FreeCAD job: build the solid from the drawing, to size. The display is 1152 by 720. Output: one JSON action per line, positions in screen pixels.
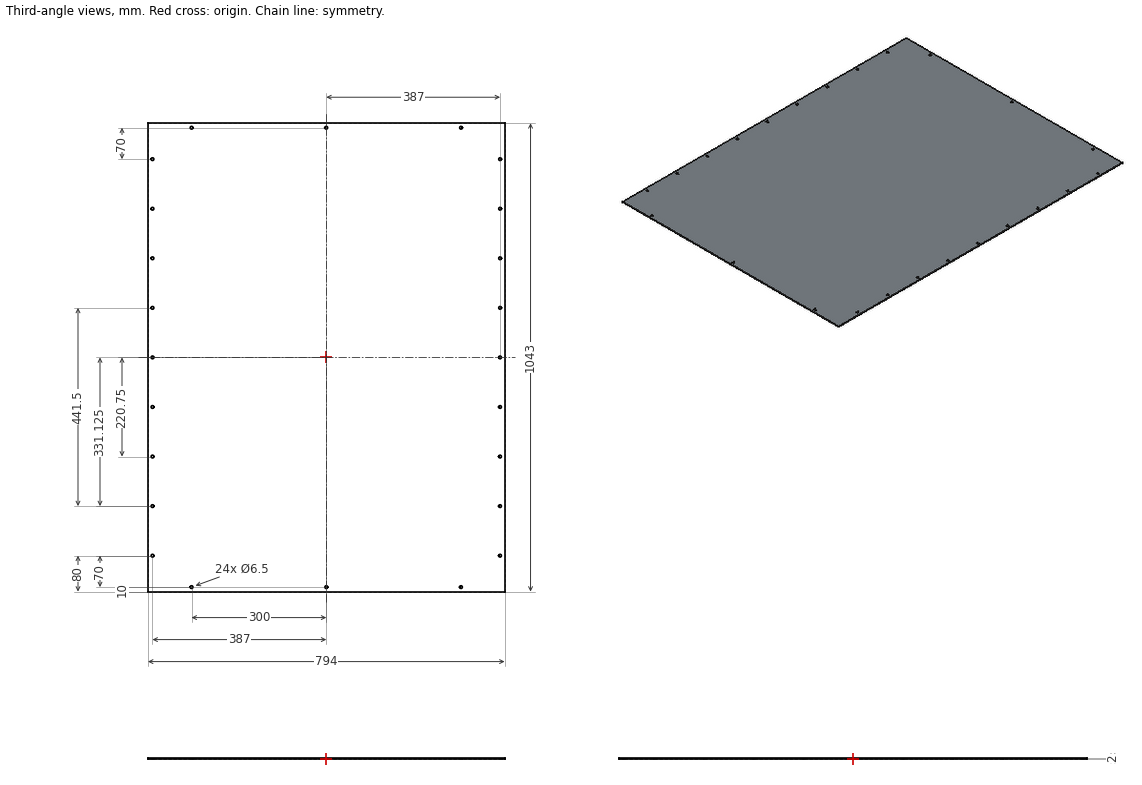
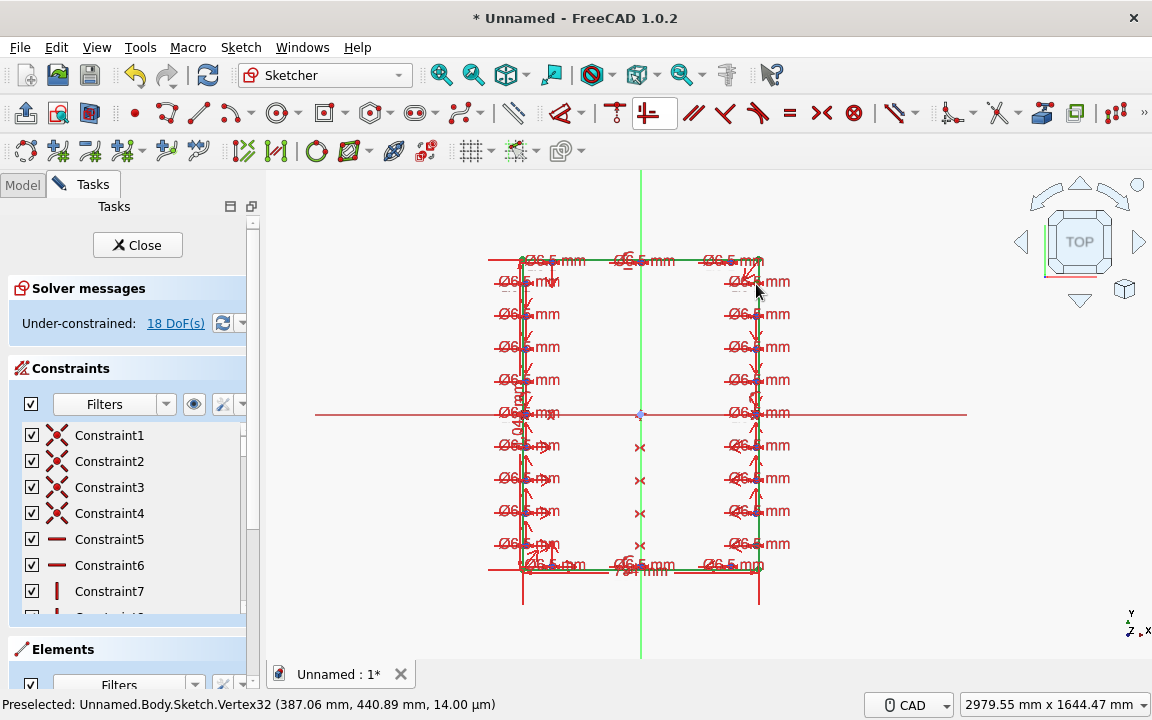
{"action": "left_click", "coordinate": [344, 415]}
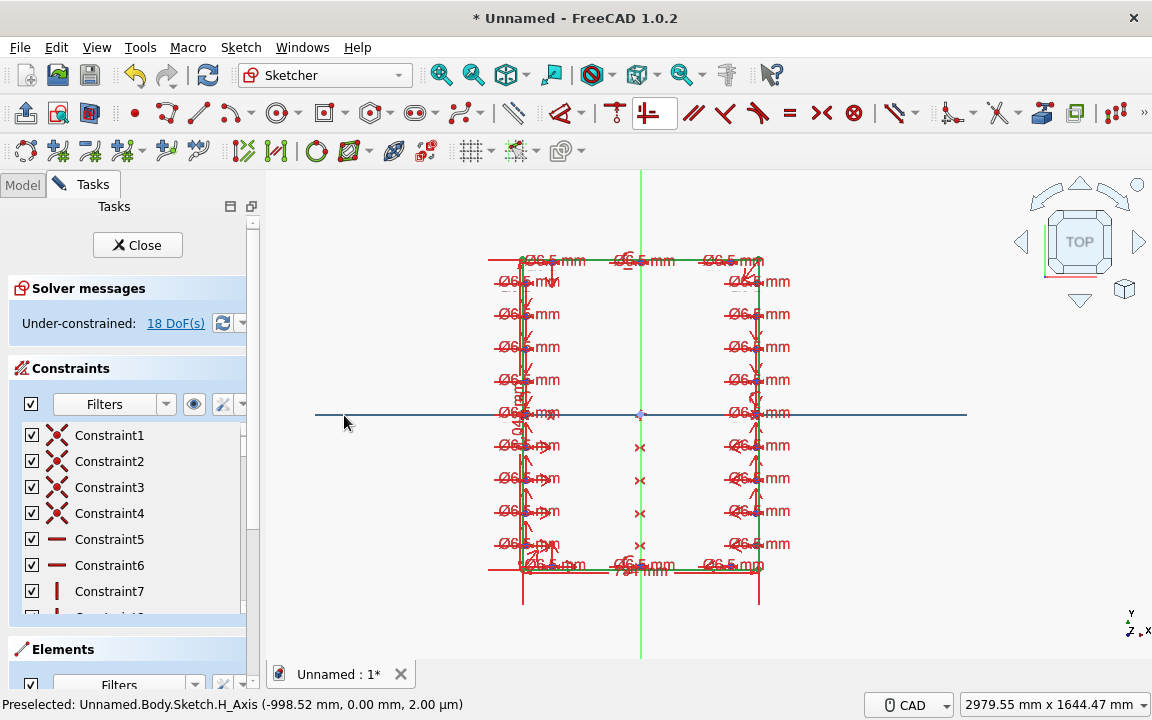
{"action": "left_click", "coordinate": [822, 114]}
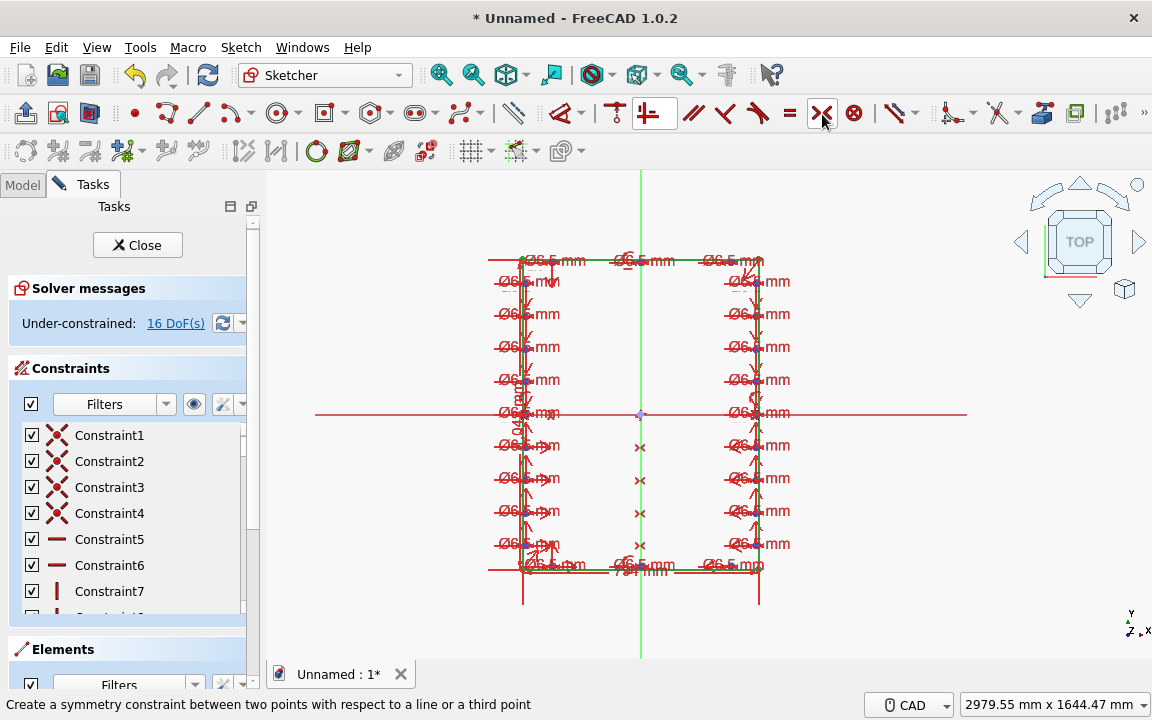
{"action": "left_click", "coordinate": [730, 567]}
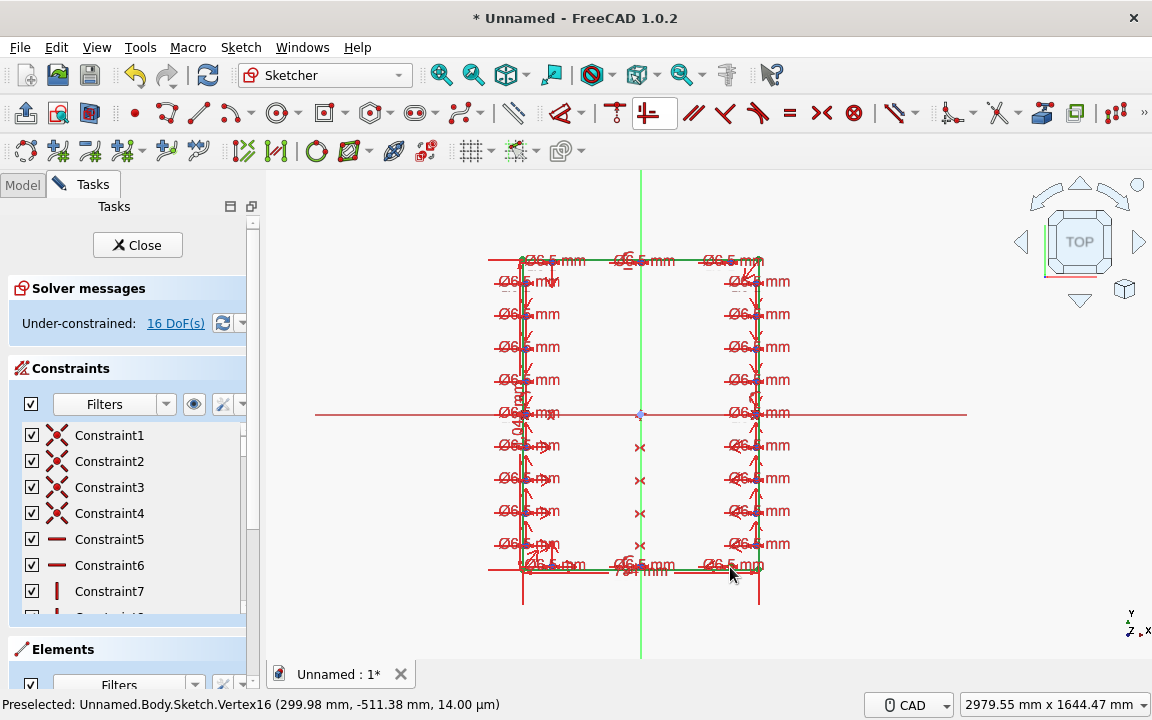
{"action": "left_click", "coordinate": [730, 263]}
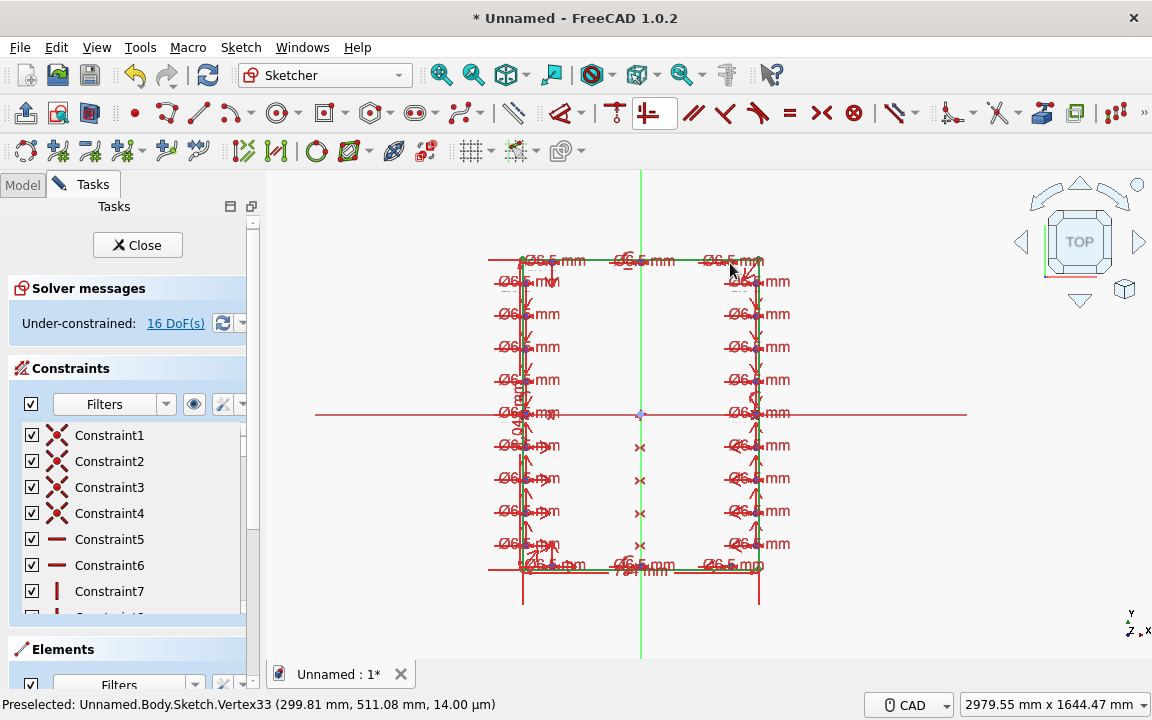
{"action": "left_click", "coordinate": [344, 415]}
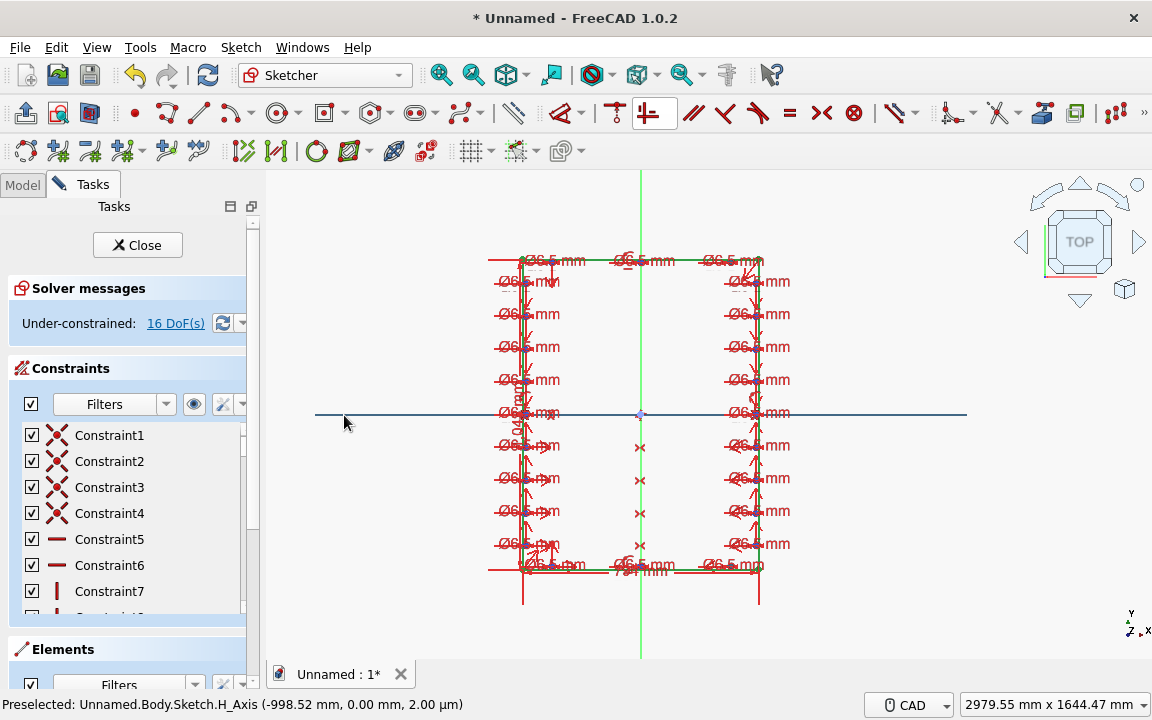
{"action": "left_click", "coordinate": [822, 114]}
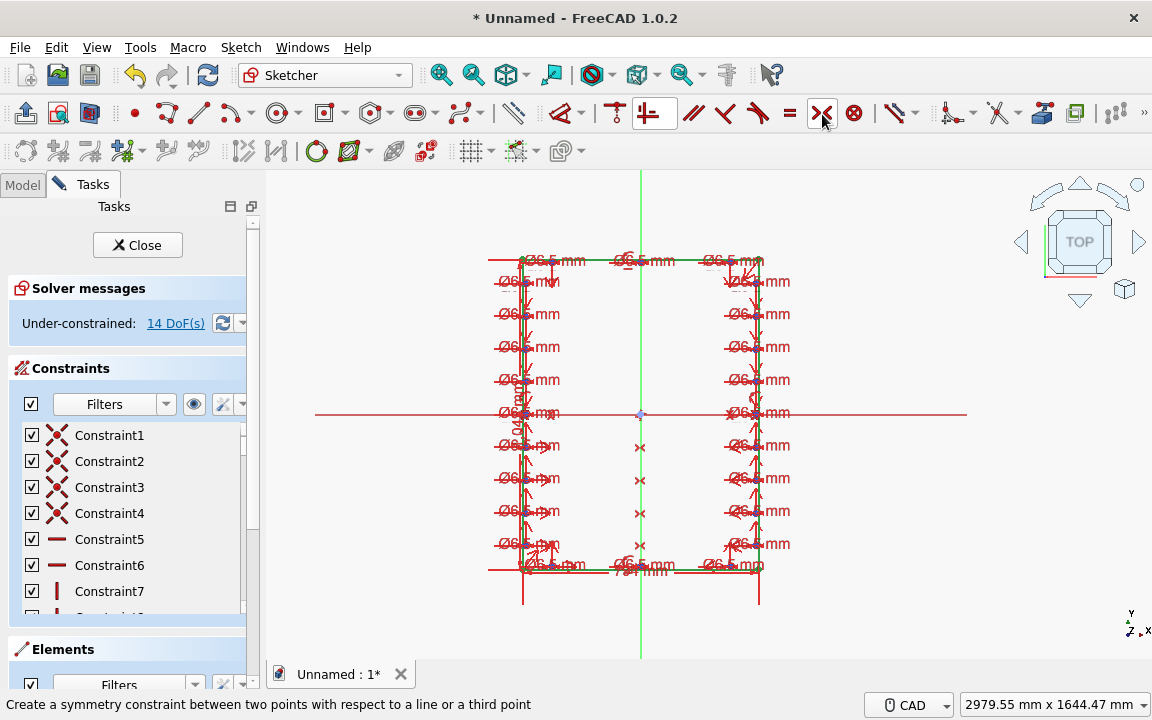
{"action": "left_click", "coordinate": [560, 114]}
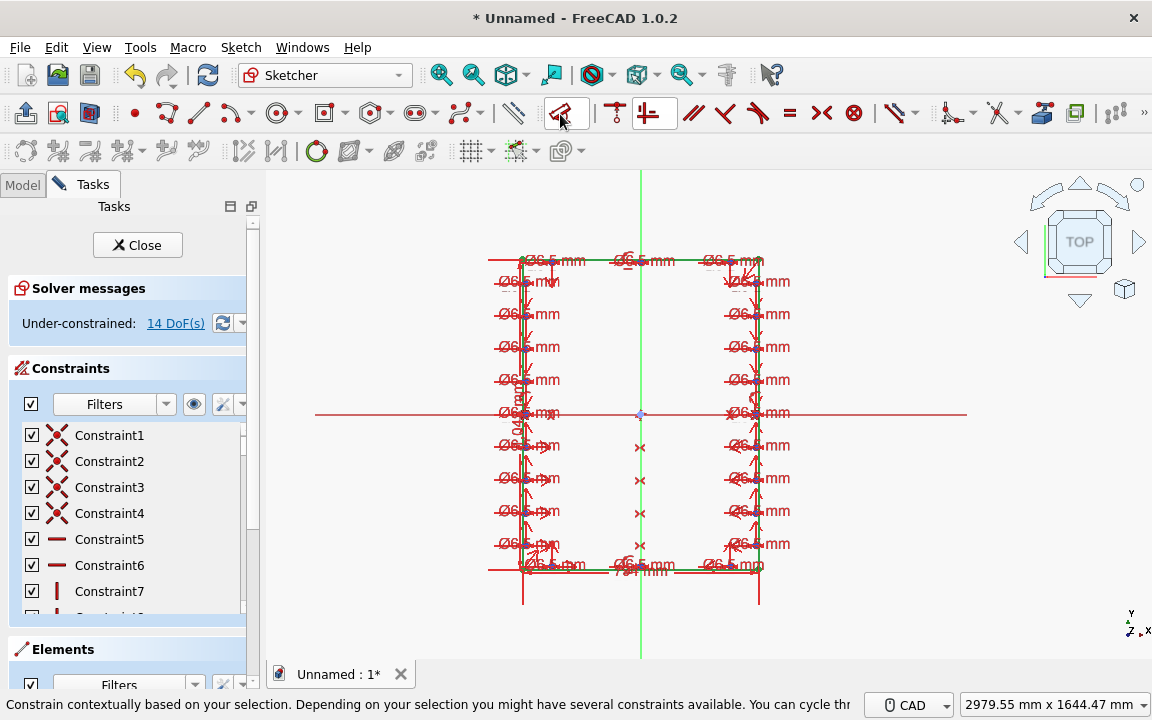
{"action": "left_click", "coordinate": [552, 567]}
{"action": "left_click", "coordinate": [596, 601]}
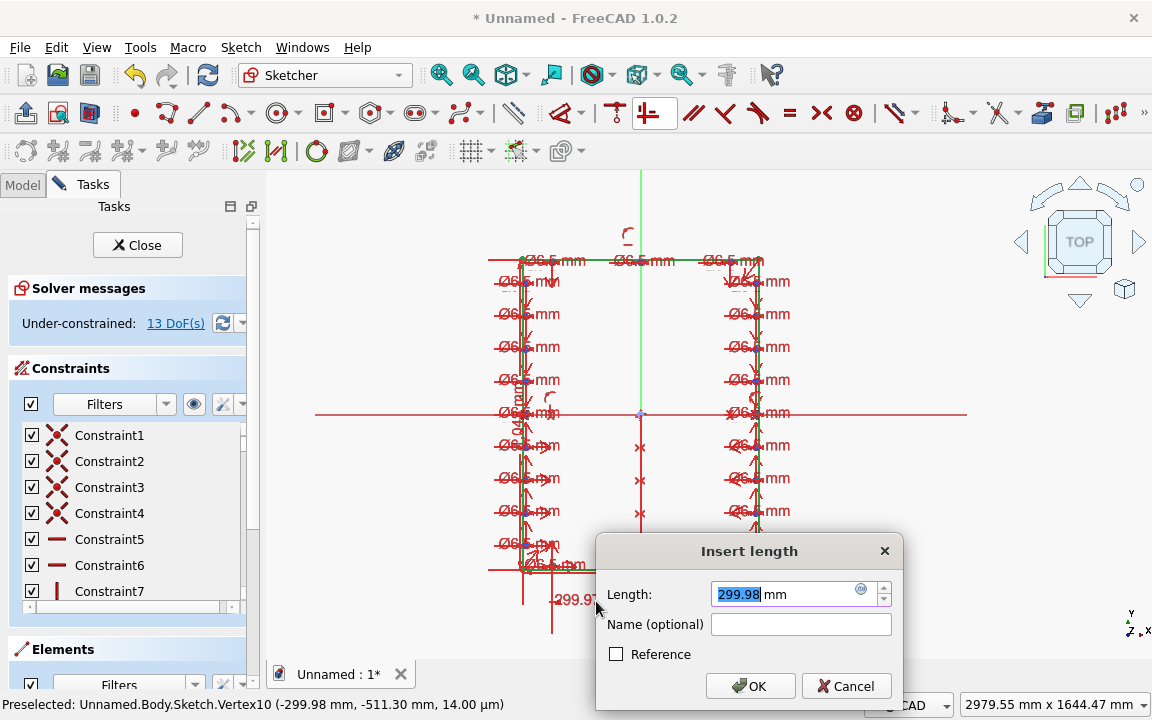
{"action": "type", "text": "300"}
{"action": "key", "text": "Return"}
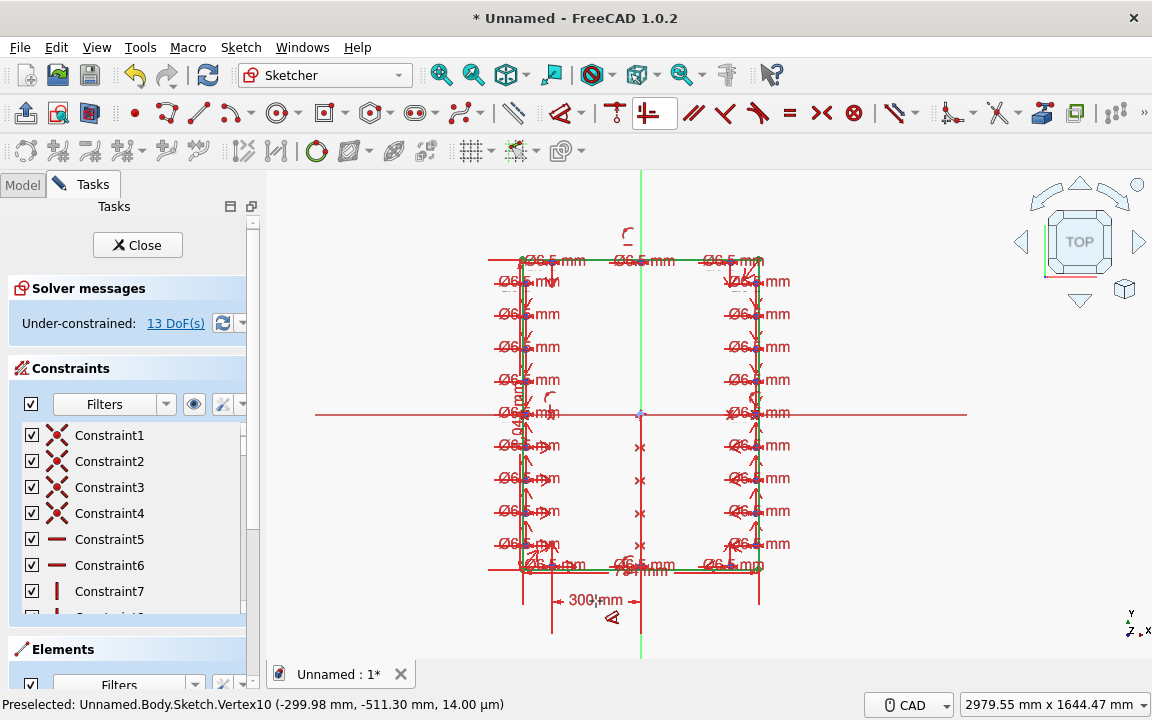
{"action": "left_click", "coordinate": [526, 546]}
{"action": "left_click", "coordinate": [583, 381]}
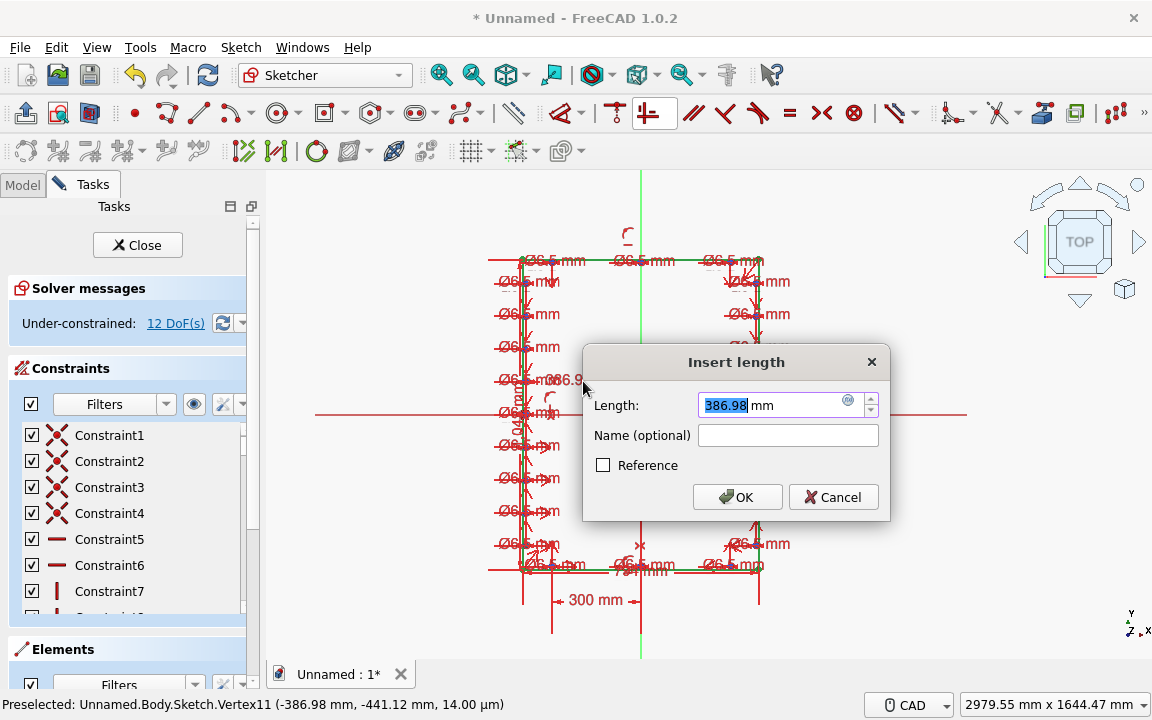
{"action": "type", "text": "387"}
{"action": "key", "text": "Return"}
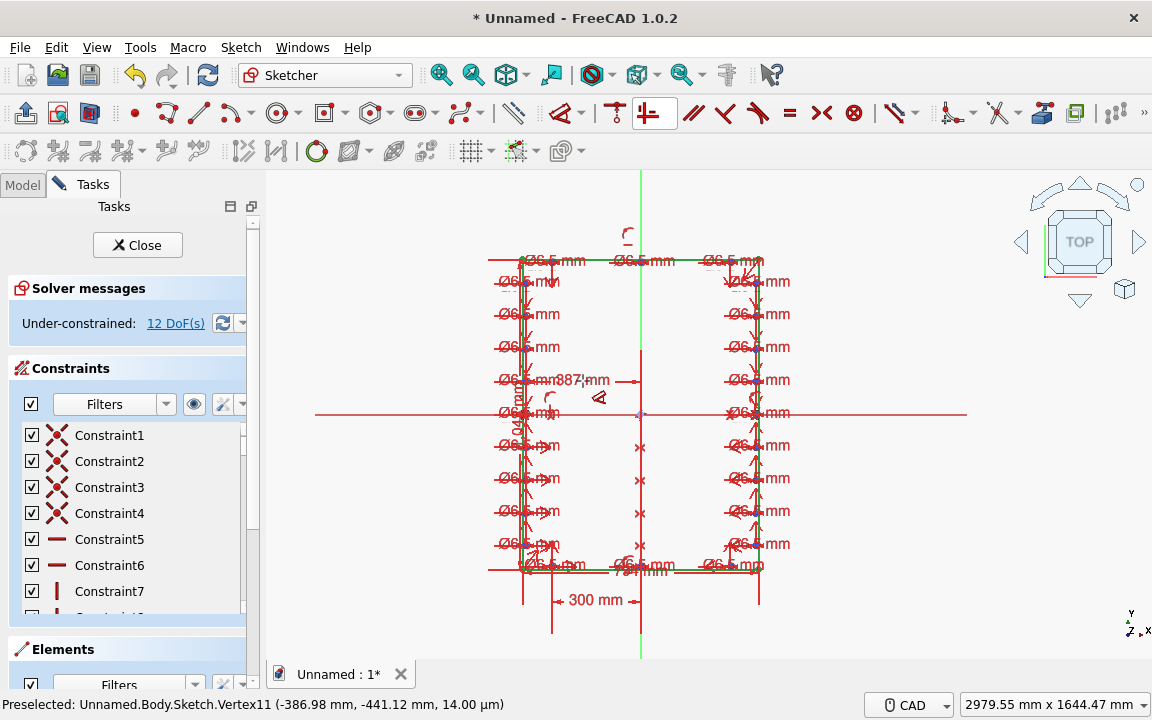
{"action": "left_click", "coordinate": [526, 513]}
{"action": "left_click", "coordinate": [583, 547]}